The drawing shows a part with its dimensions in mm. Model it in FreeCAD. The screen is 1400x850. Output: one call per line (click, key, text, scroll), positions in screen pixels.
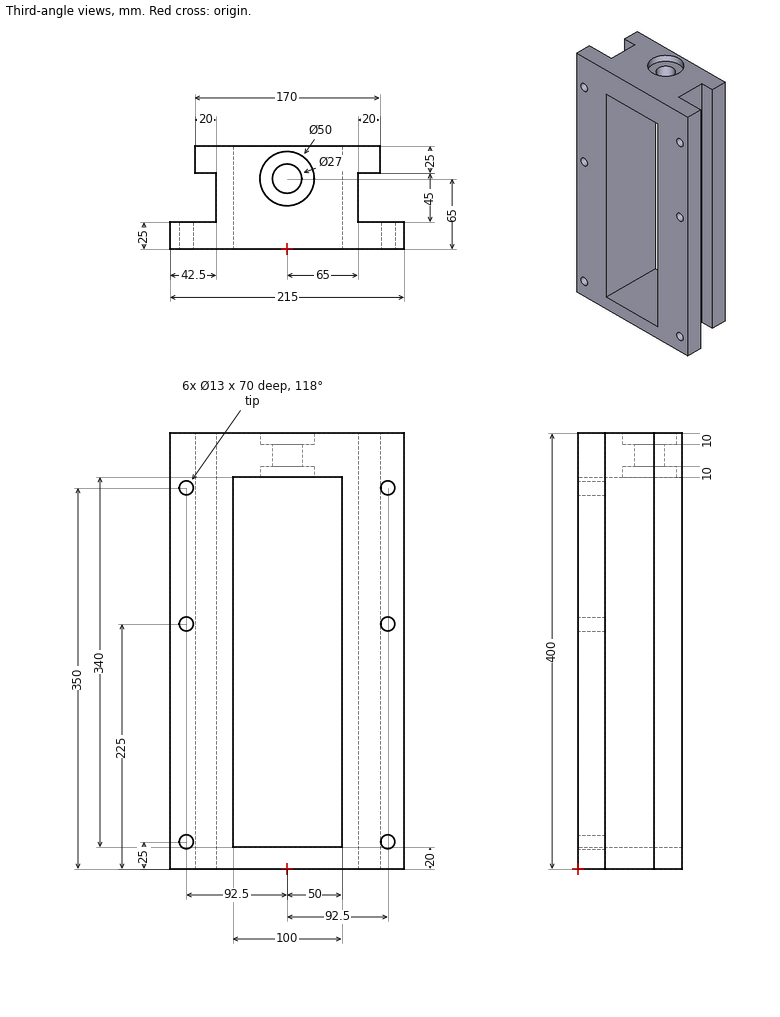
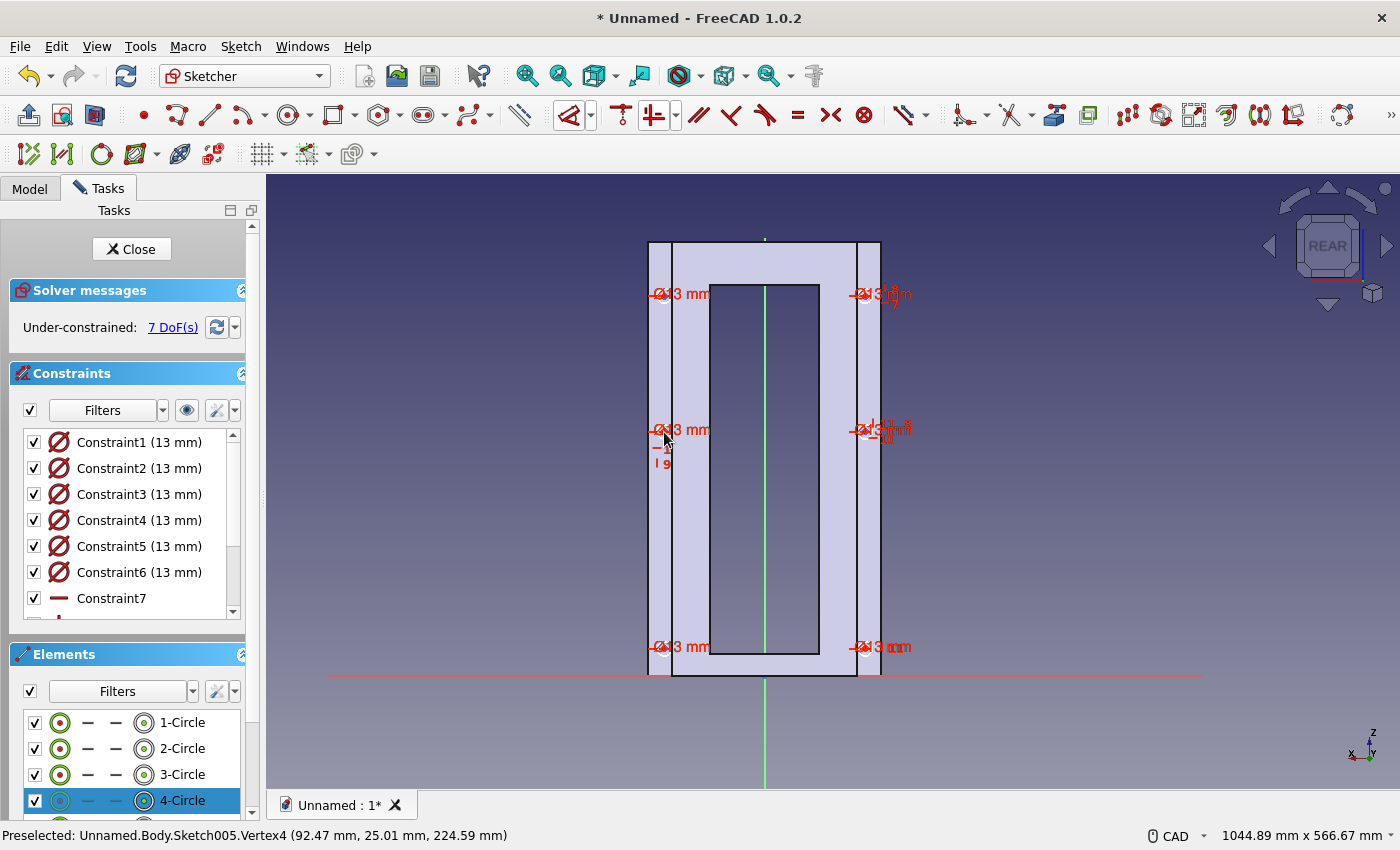
click(664, 649)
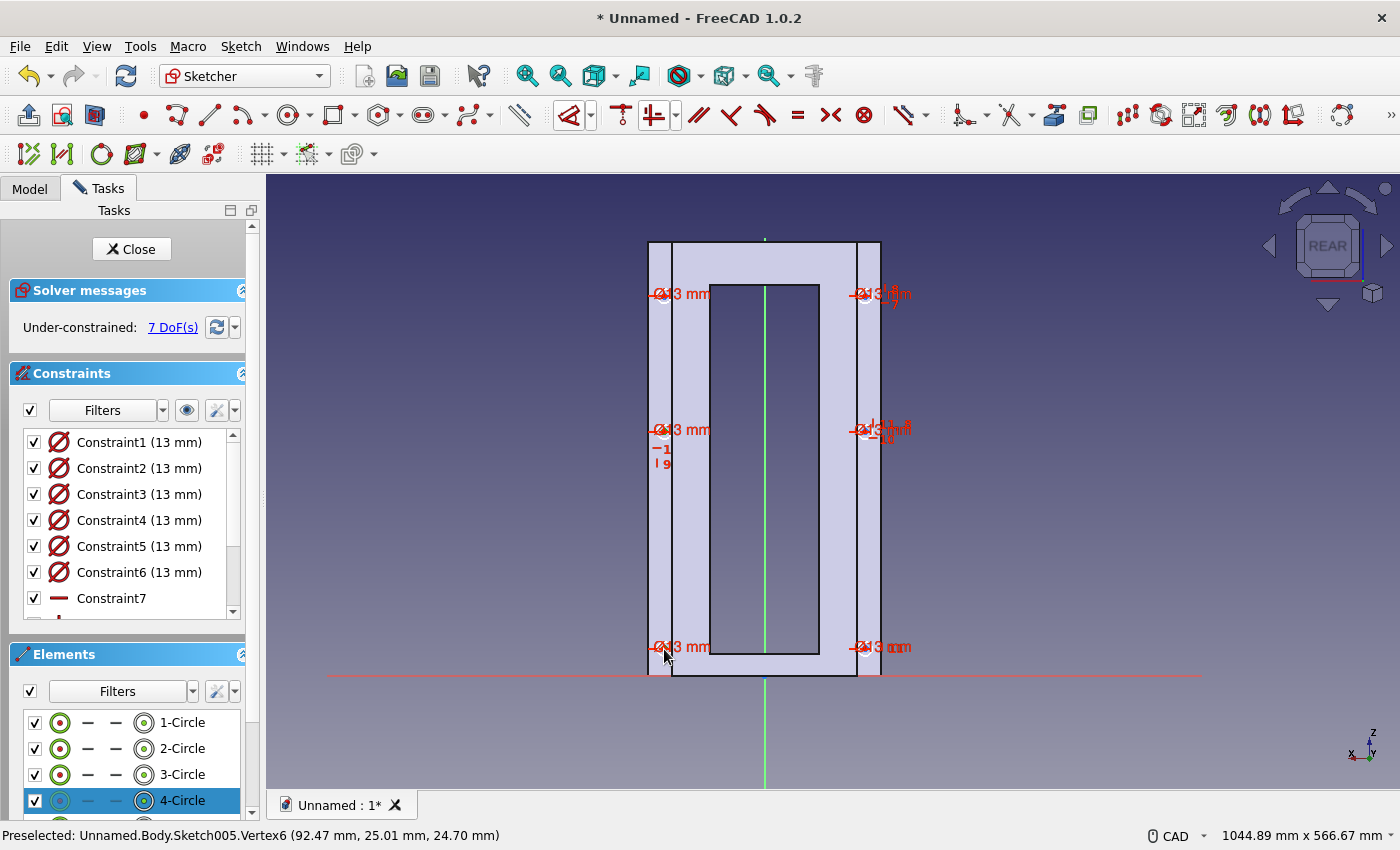
key(v)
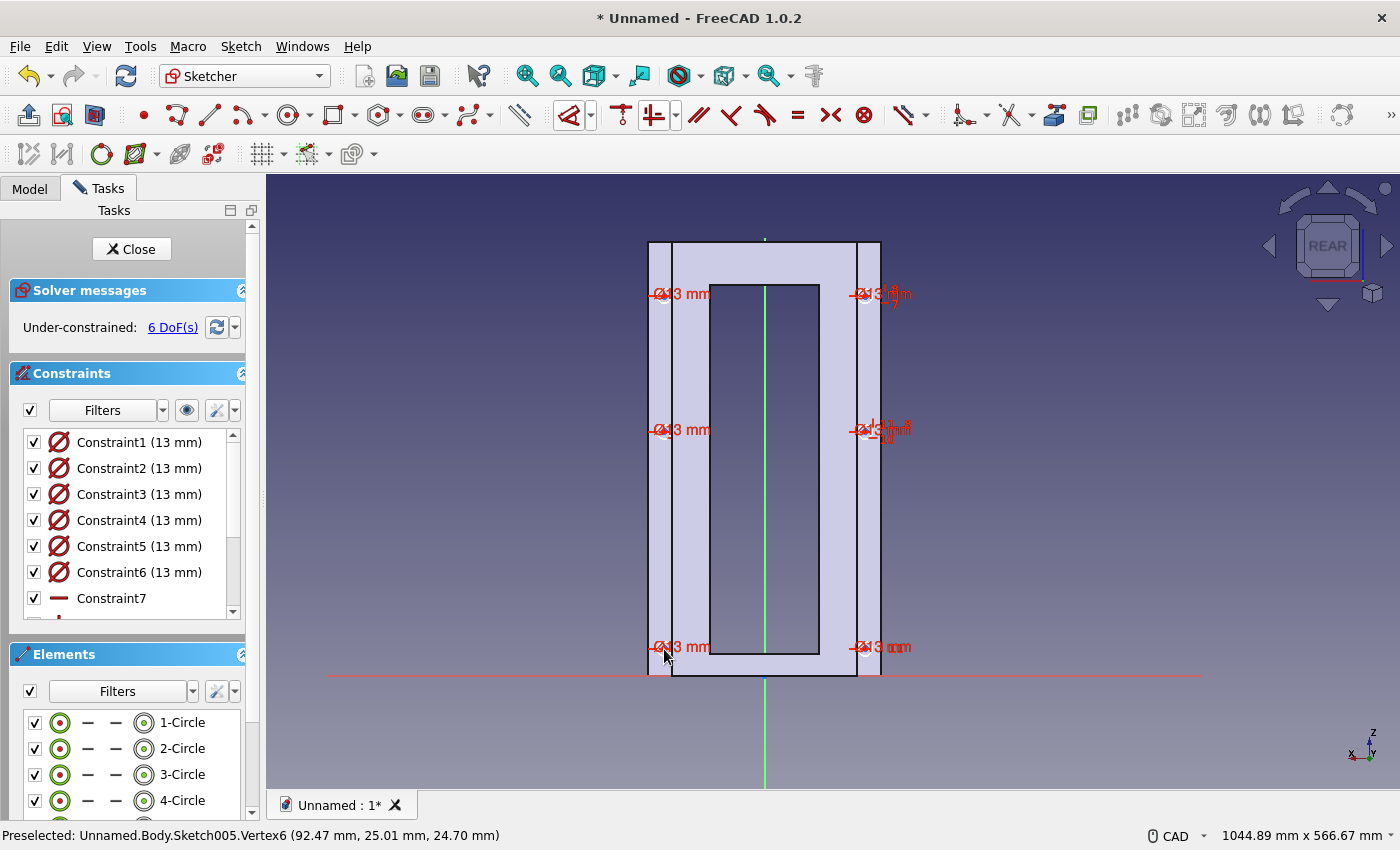
click(865, 649)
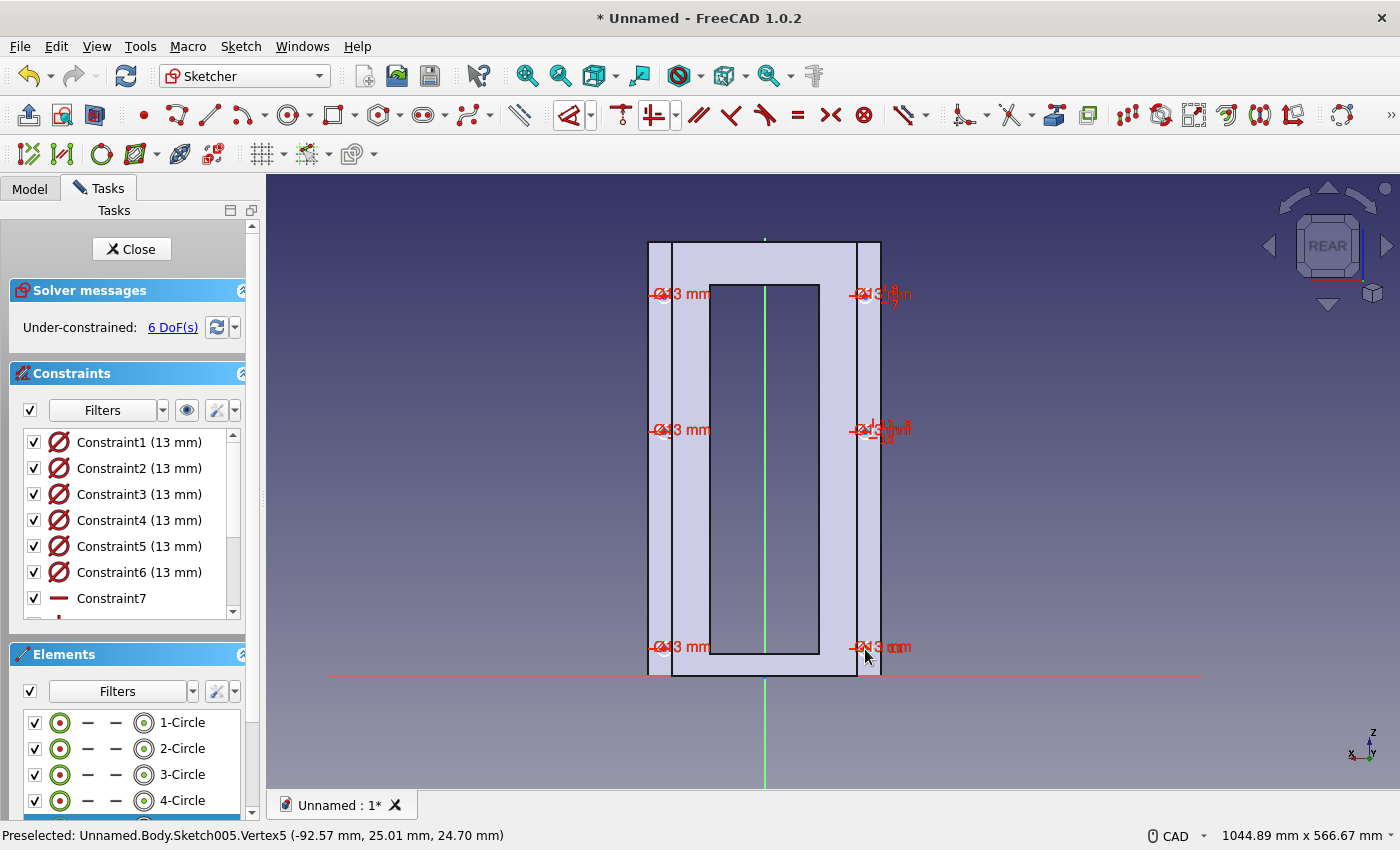
click(664, 649)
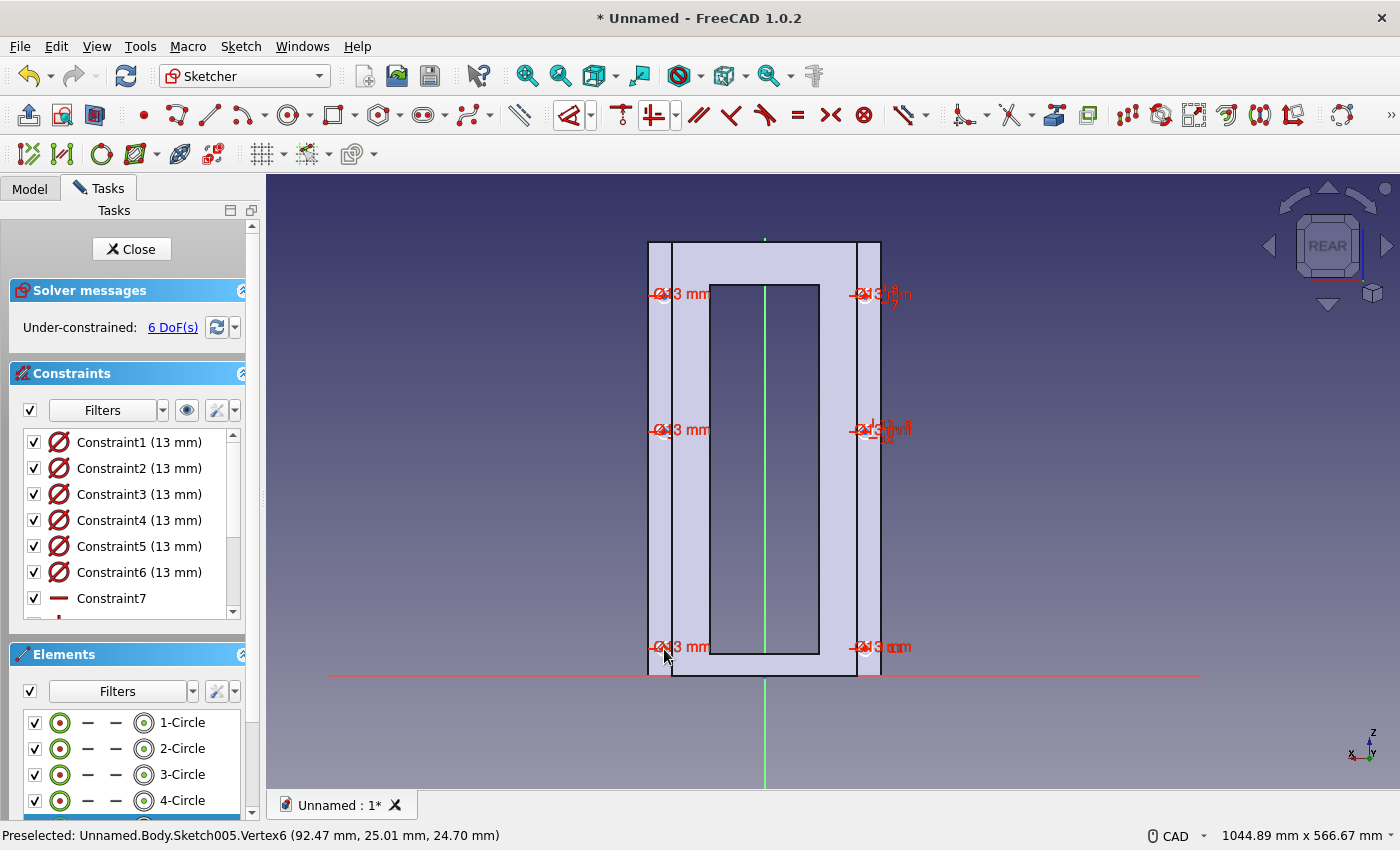
click(676, 116)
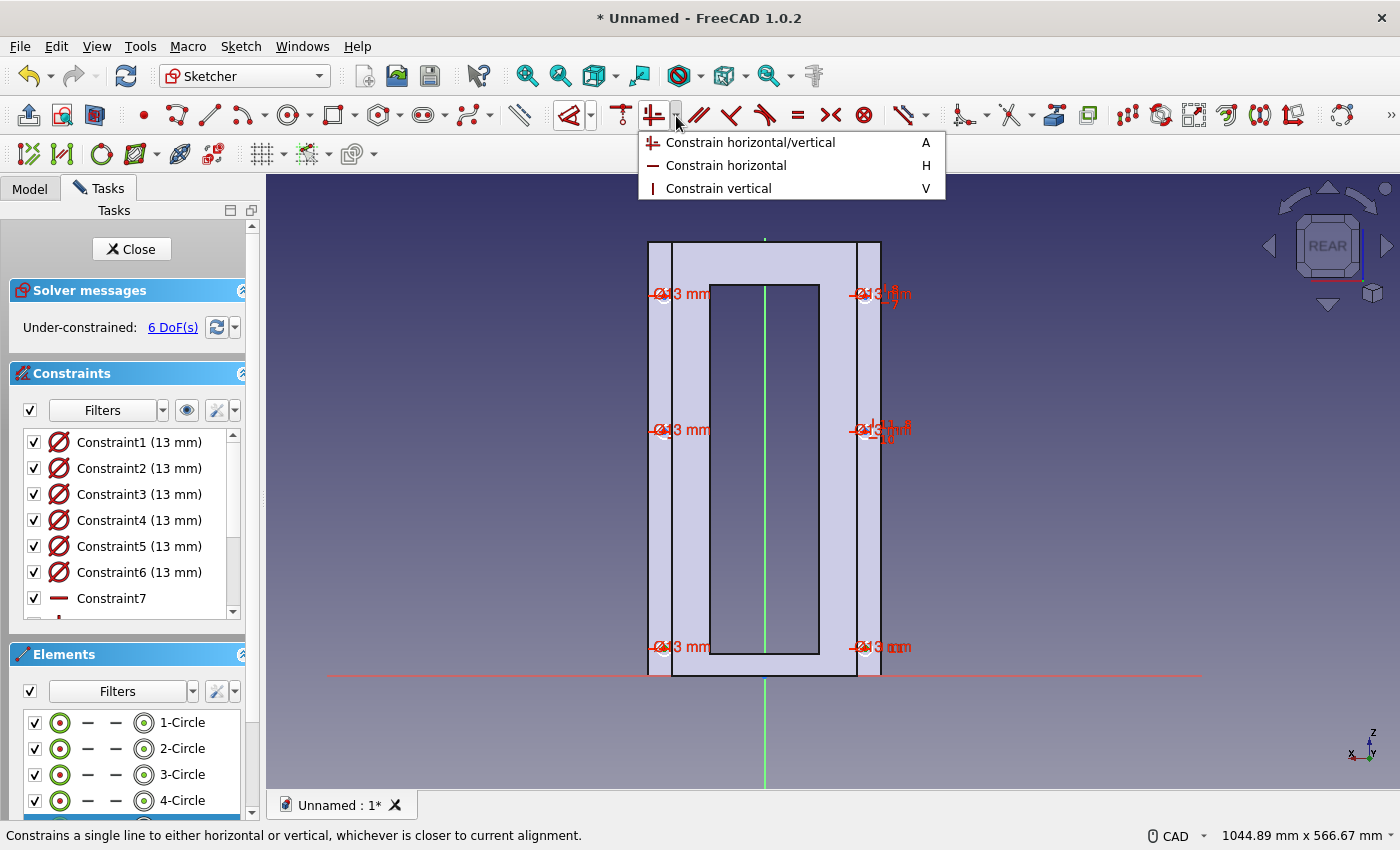
click(792, 166)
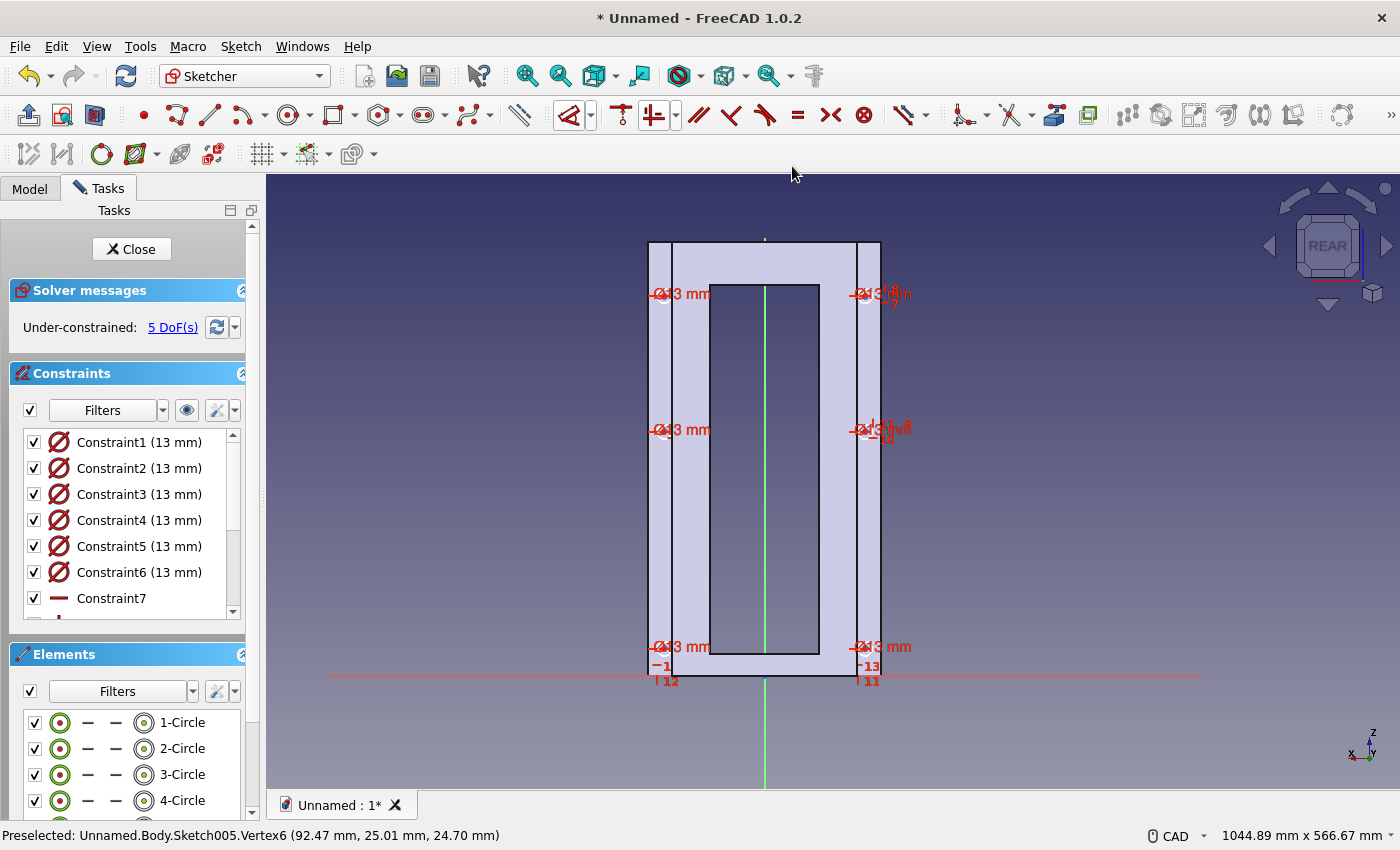
scroll(865, 649, up, 2)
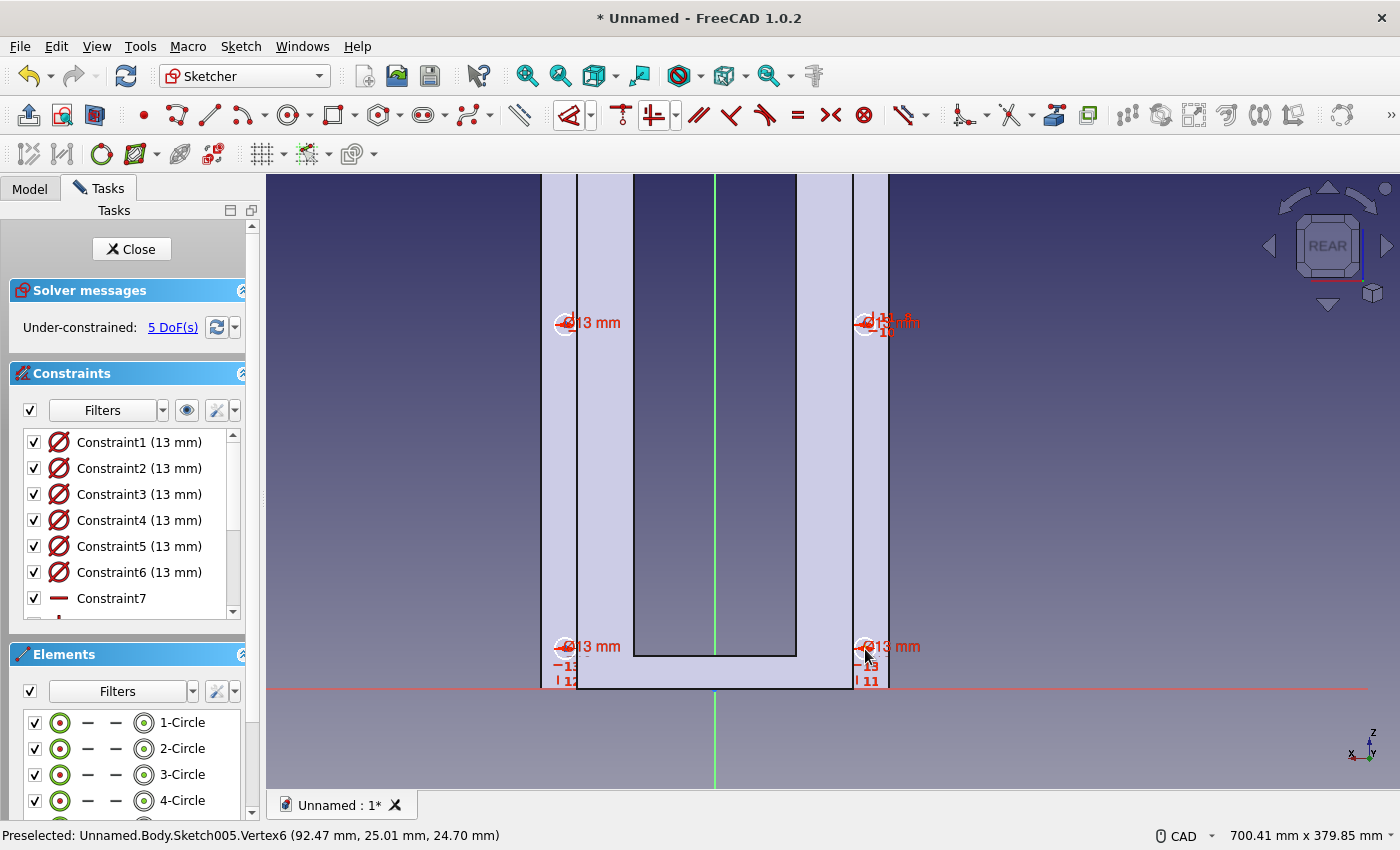
click(865, 649)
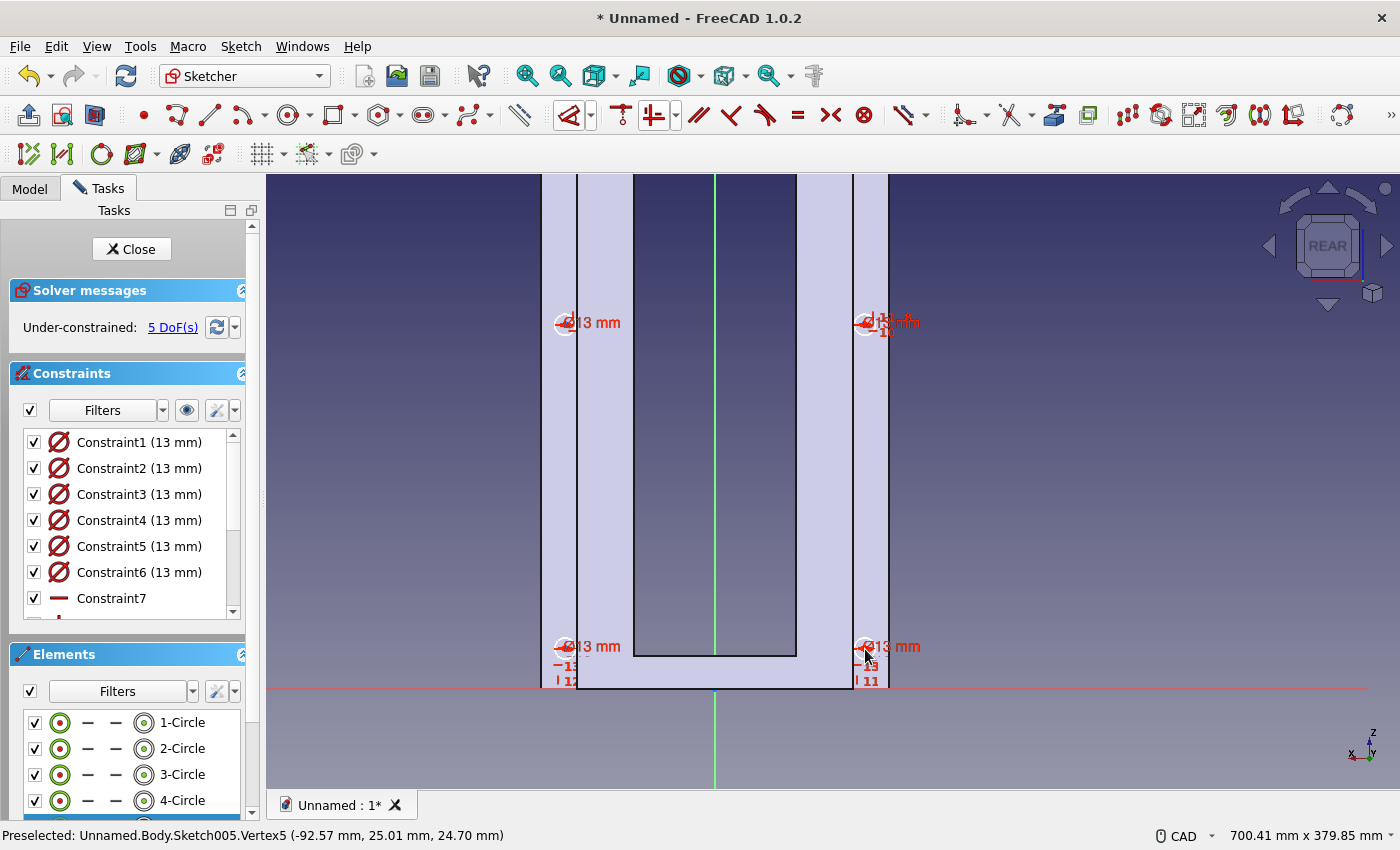
key(i)